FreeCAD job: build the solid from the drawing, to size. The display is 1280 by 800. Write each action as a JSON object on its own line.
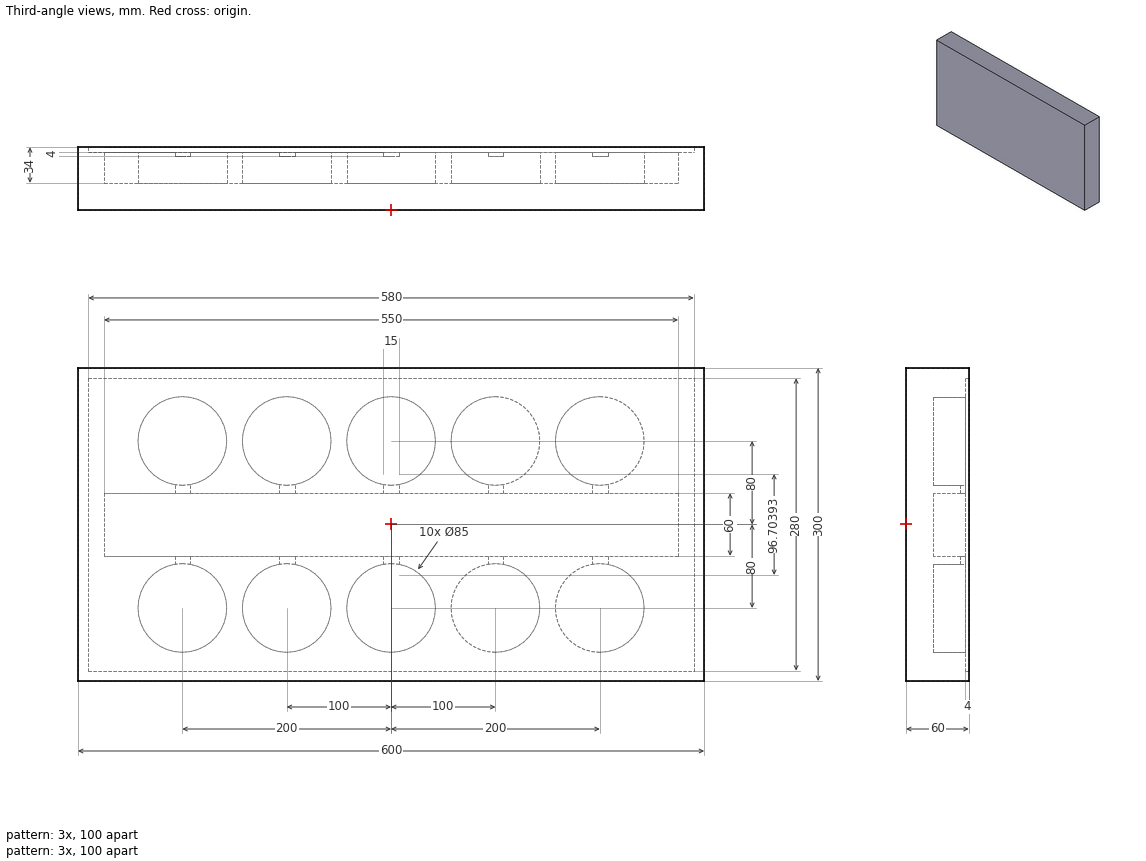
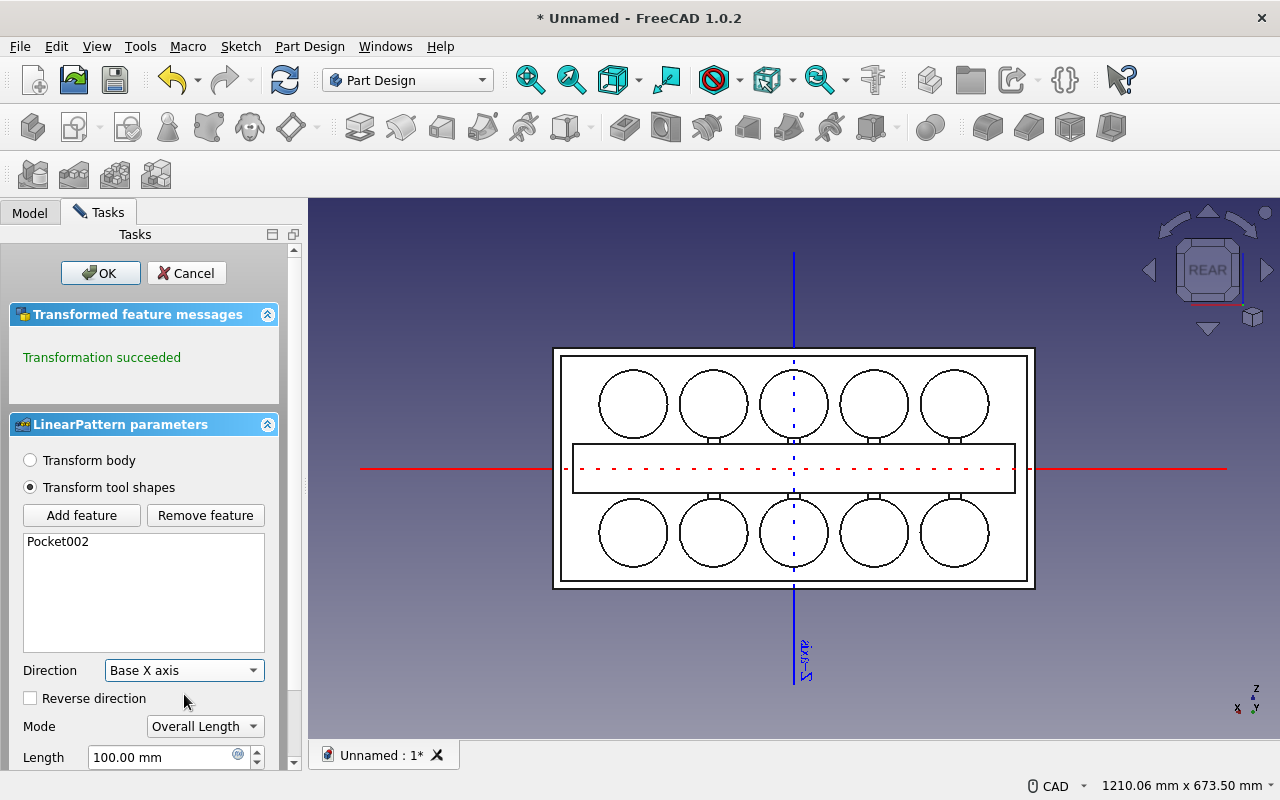
{"action": "left_click", "coordinate": [206, 726]}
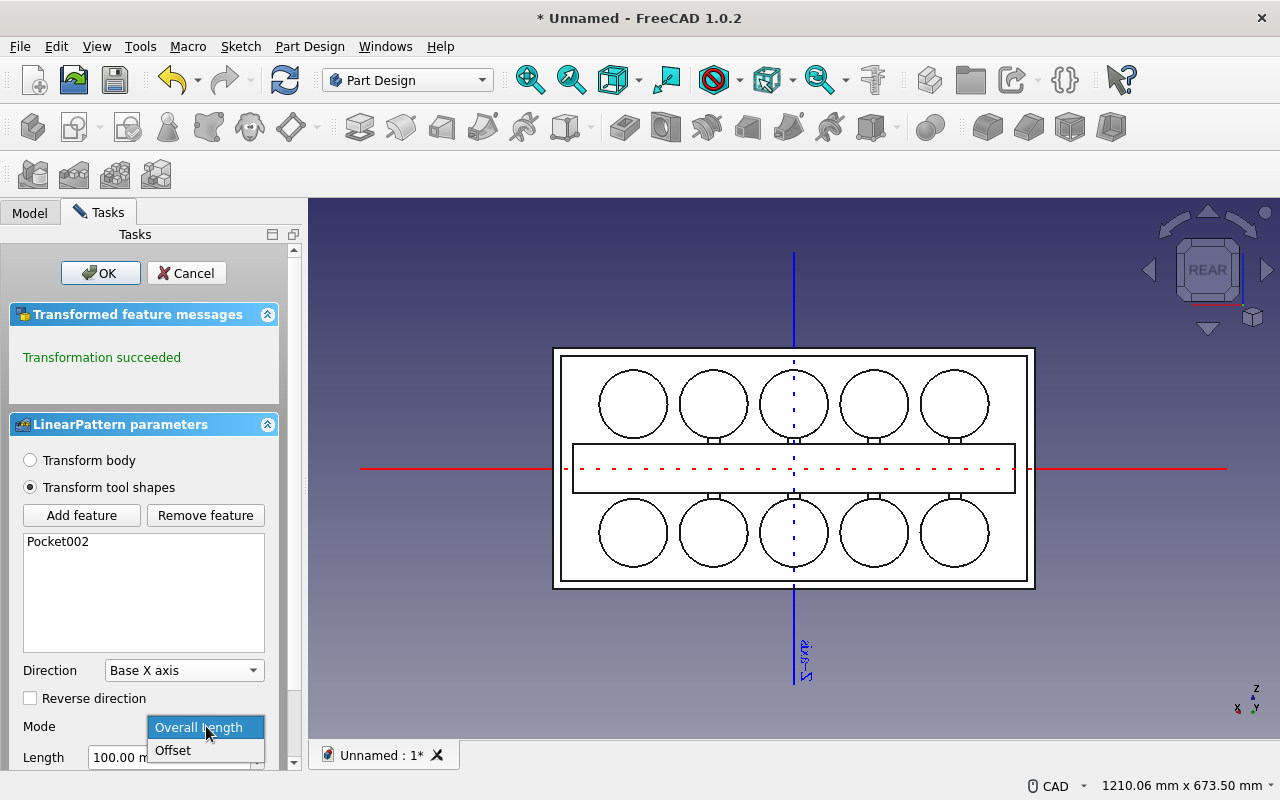
{"action": "left_click", "coordinate": [204, 750]}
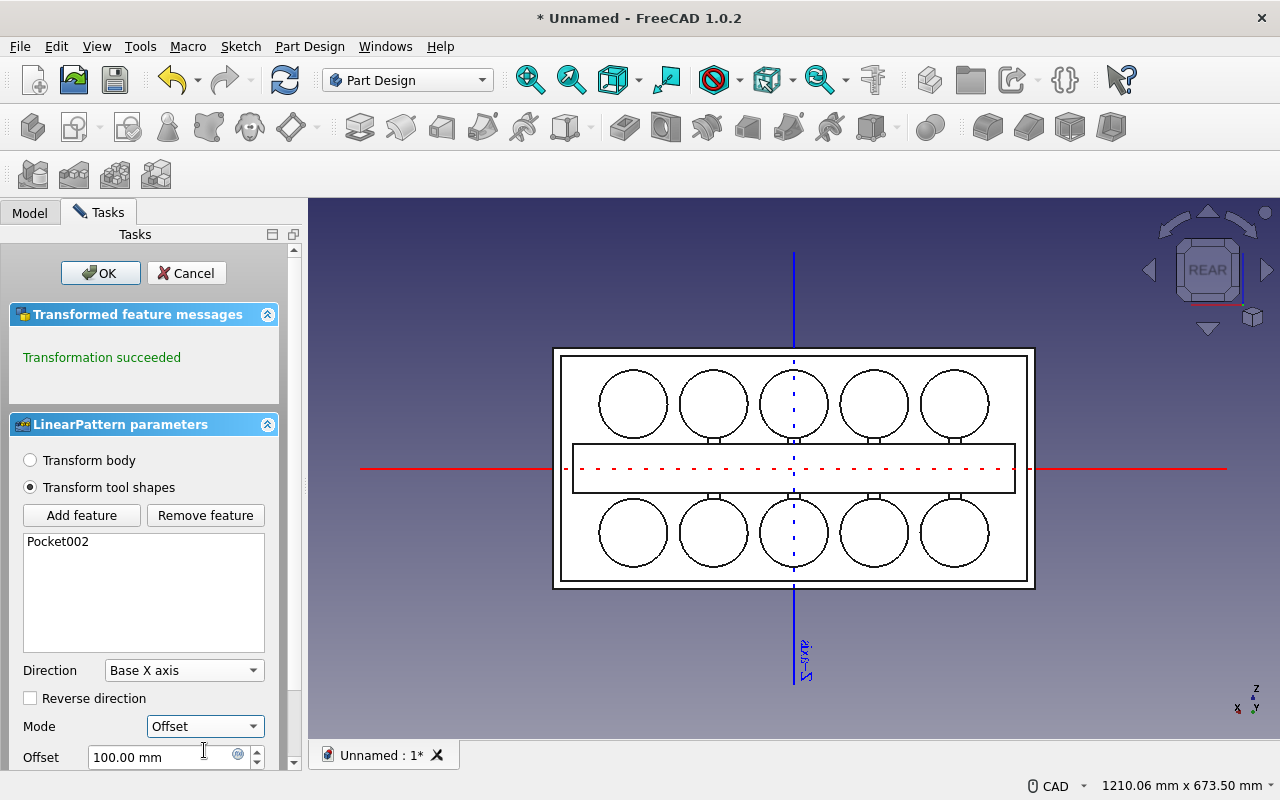
{"action": "scroll", "coordinate": [294, 507], "scroll_direction": "down", "scroll_amount": 2}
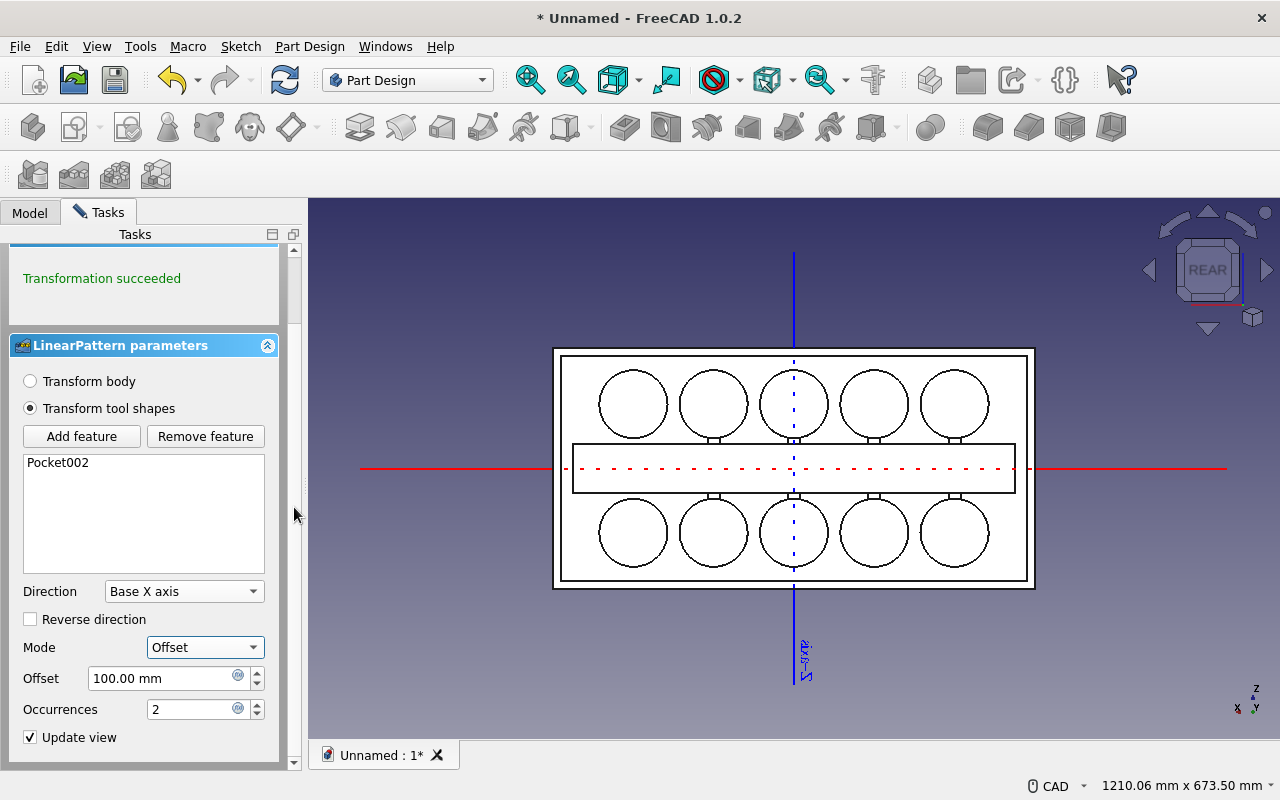
{"action": "triple_click", "coordinate": [170, 678]}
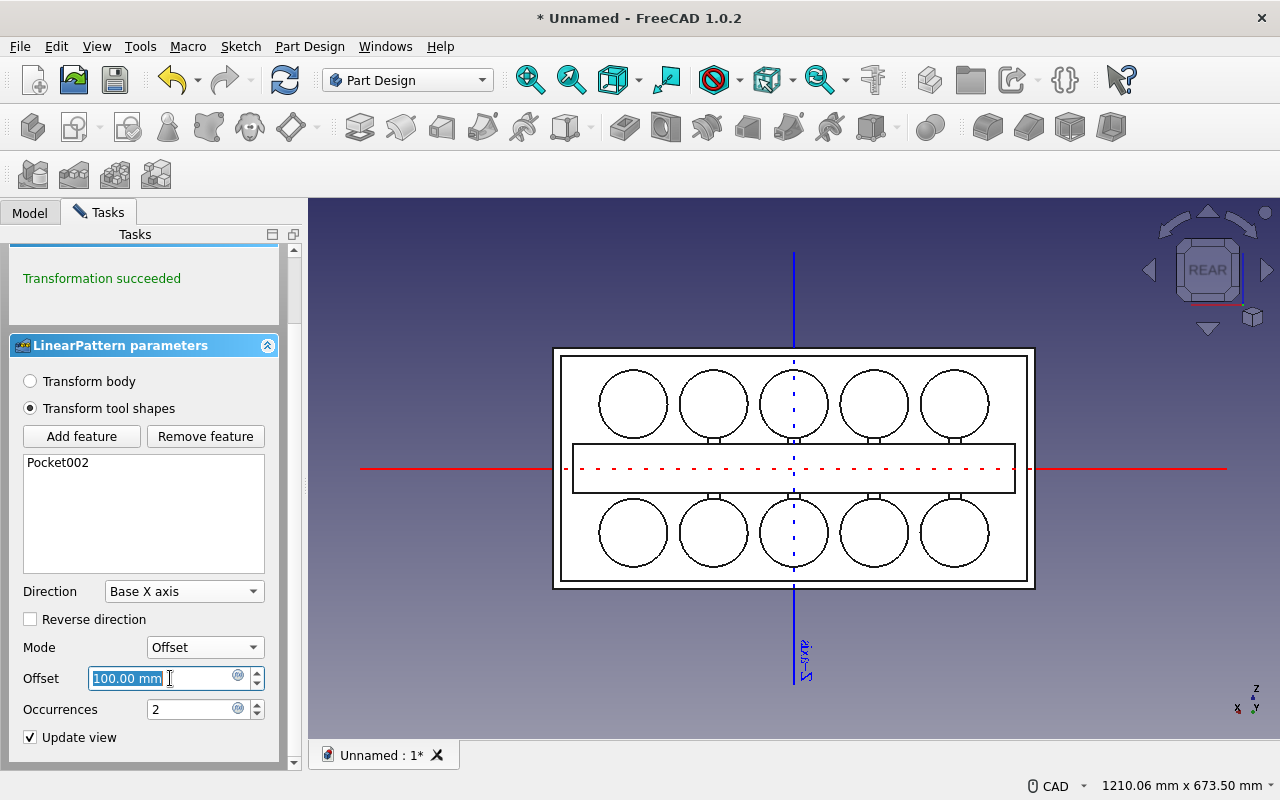
{"action": "type", "text": "100"}
{"action": "key", "text": "Tab"}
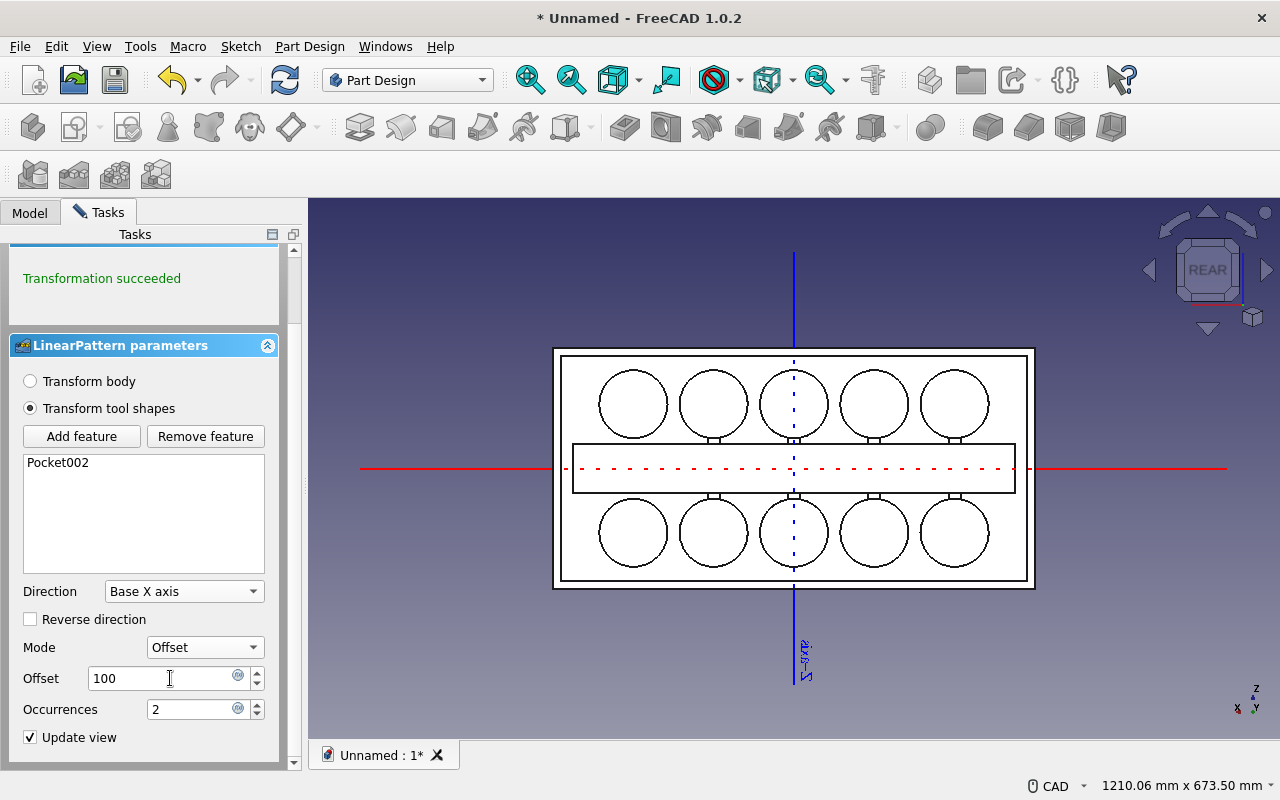
{"action": "triple_click", "coordinate": [199, 710]}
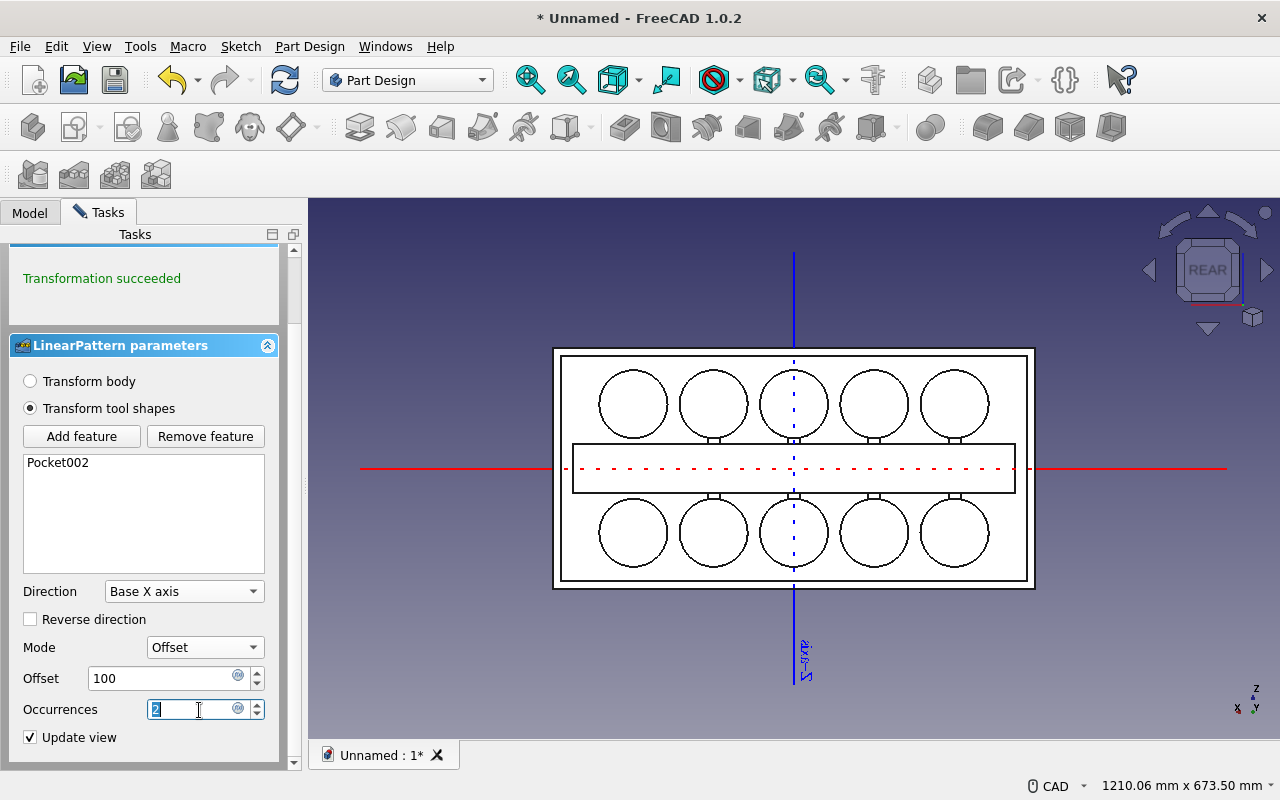
{"action": "type", "text": "3"}
{"action": "key", "text": "Tab"}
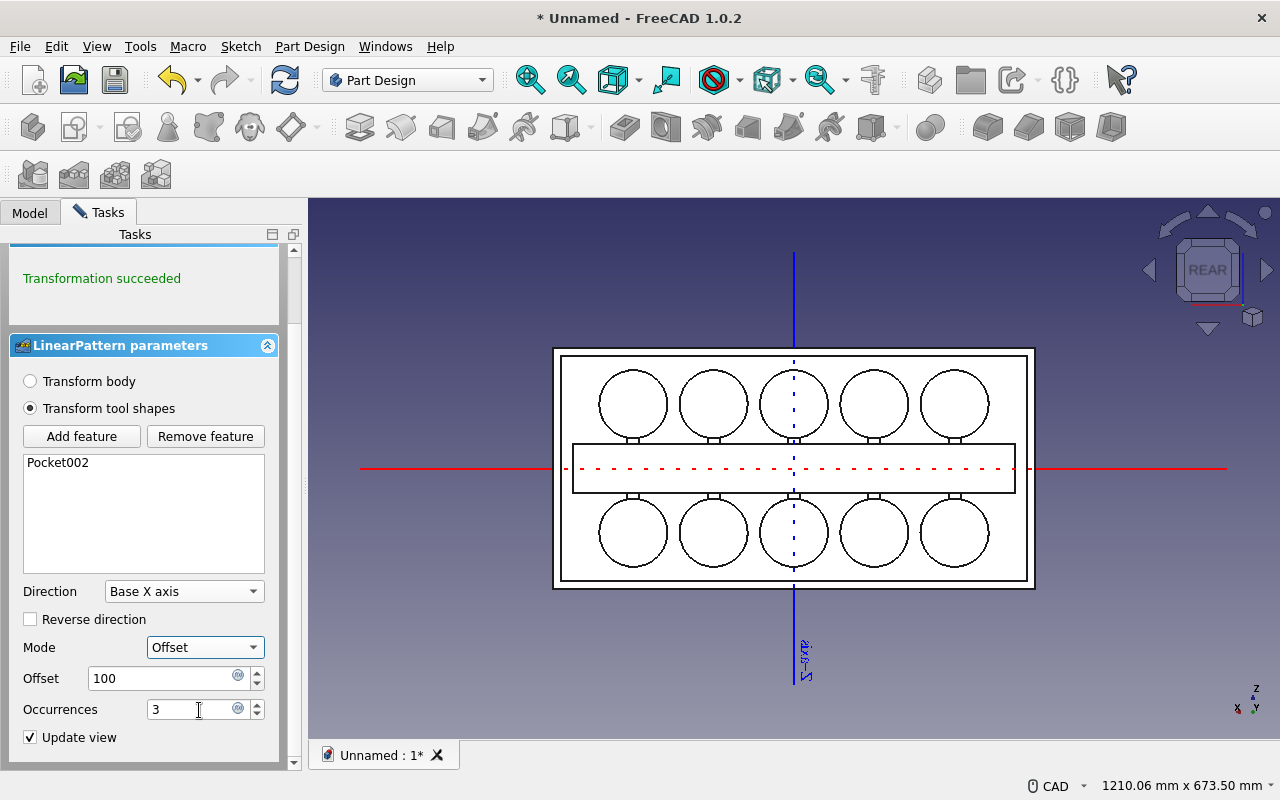
{"action": "scroll", "coordinate": [294, 507], "scroll_direction": "up", "scroll_amount": 3}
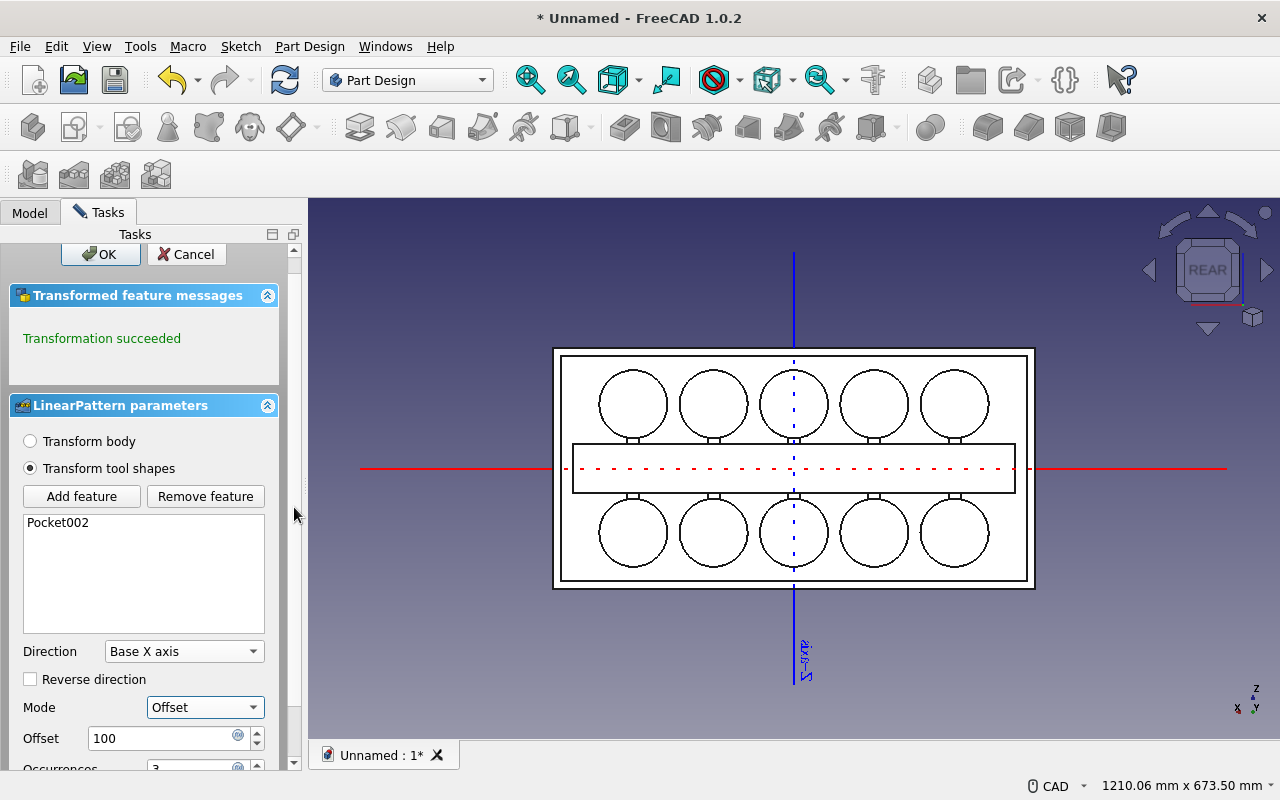
{"action": "left_click", "coordinate": [101, 273]}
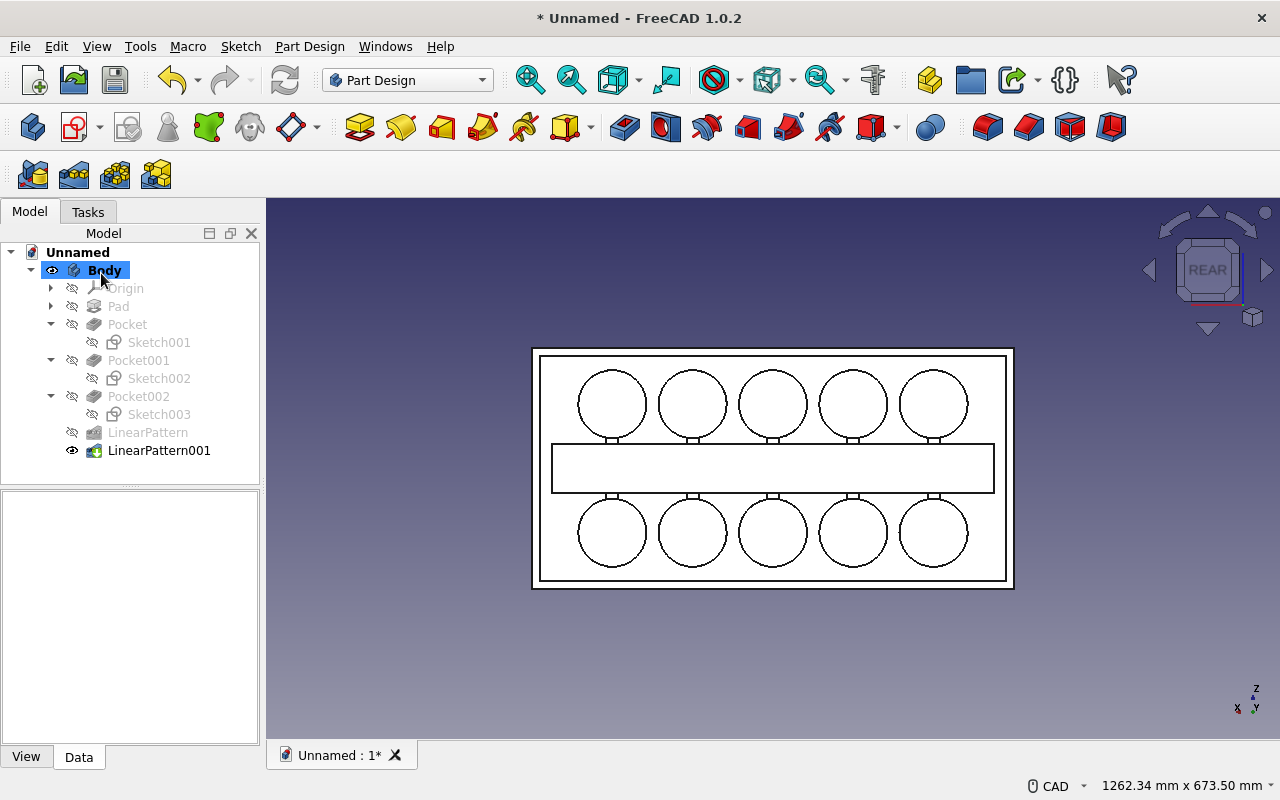
{"action": "key", "text": "0"}